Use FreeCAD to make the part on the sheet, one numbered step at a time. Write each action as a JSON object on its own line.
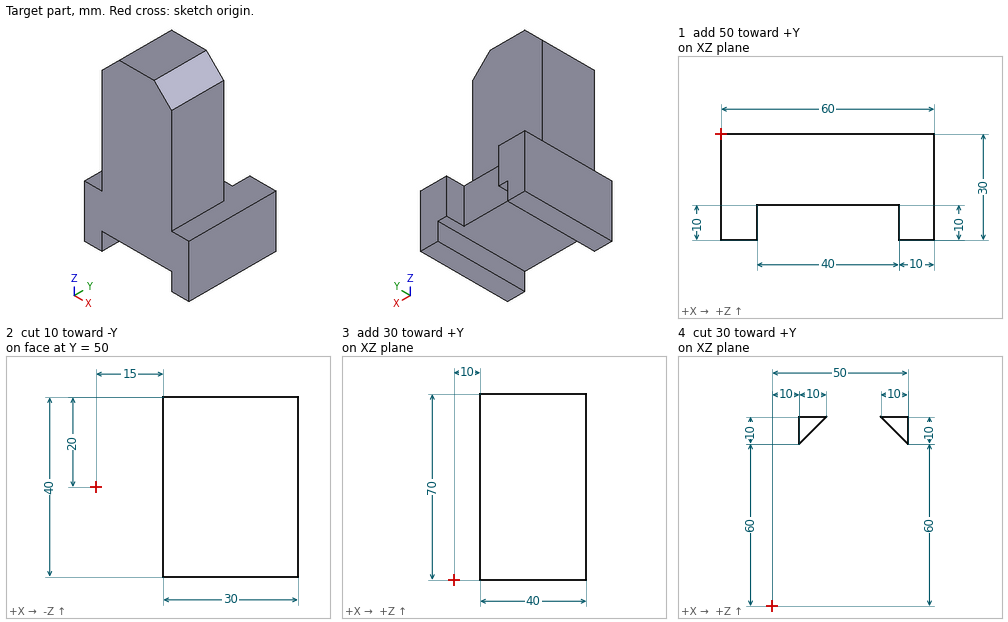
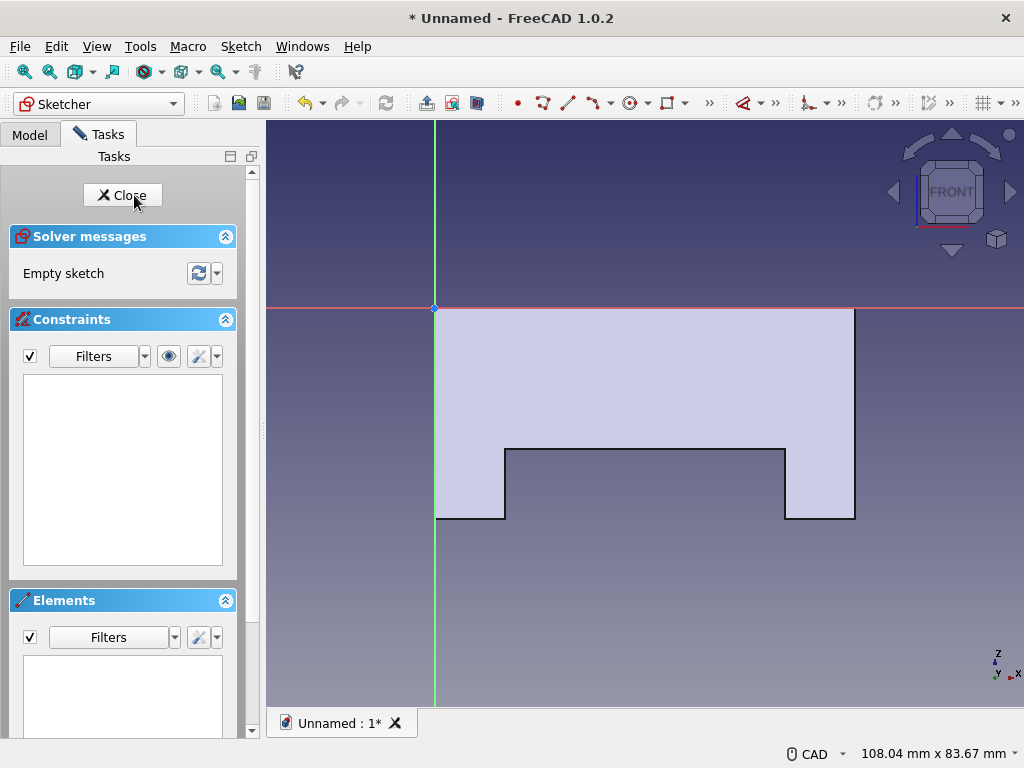
{"action": "scroll", "coordinate": [536, 679], "scroll_direction": "down", "scroll_amount": 3}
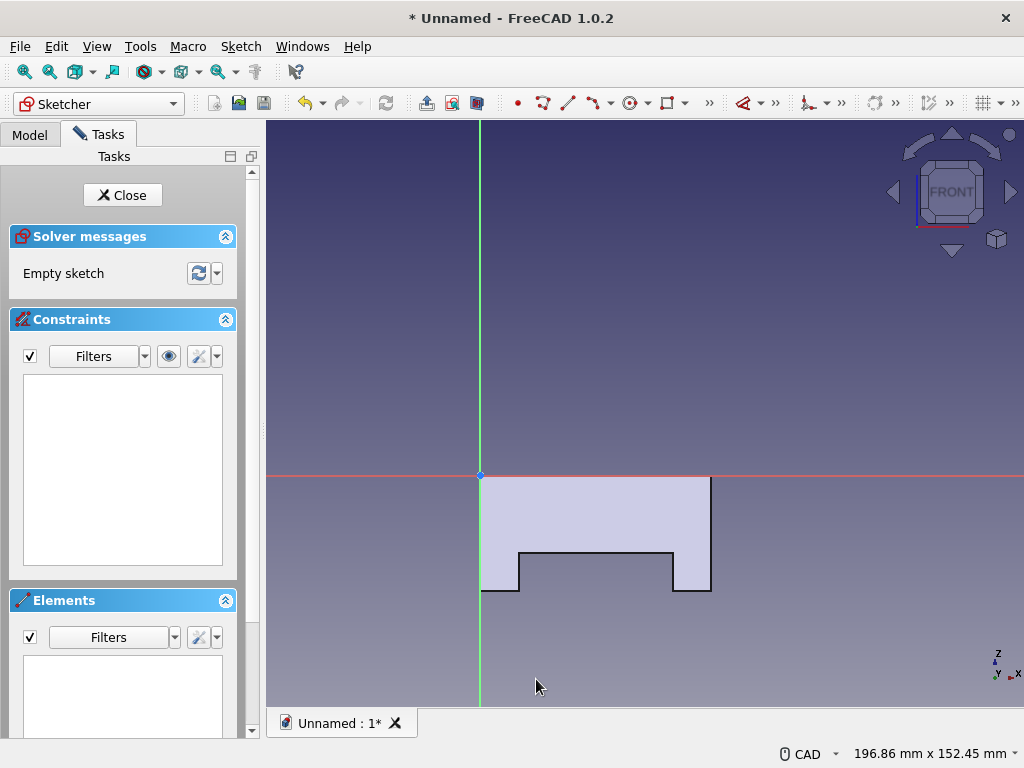
{"action": "scroll", "coordinate": [577, 194], "scroll_direction": "up", "scroll_amount": 2}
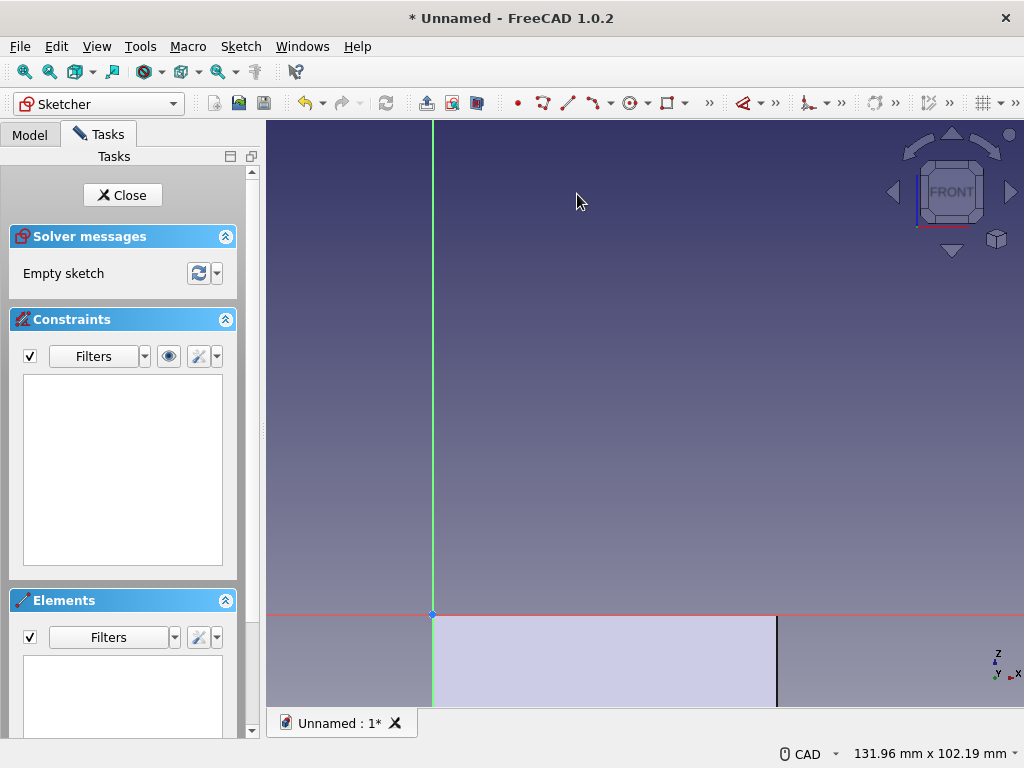
{"action": "key", "text": "g r"}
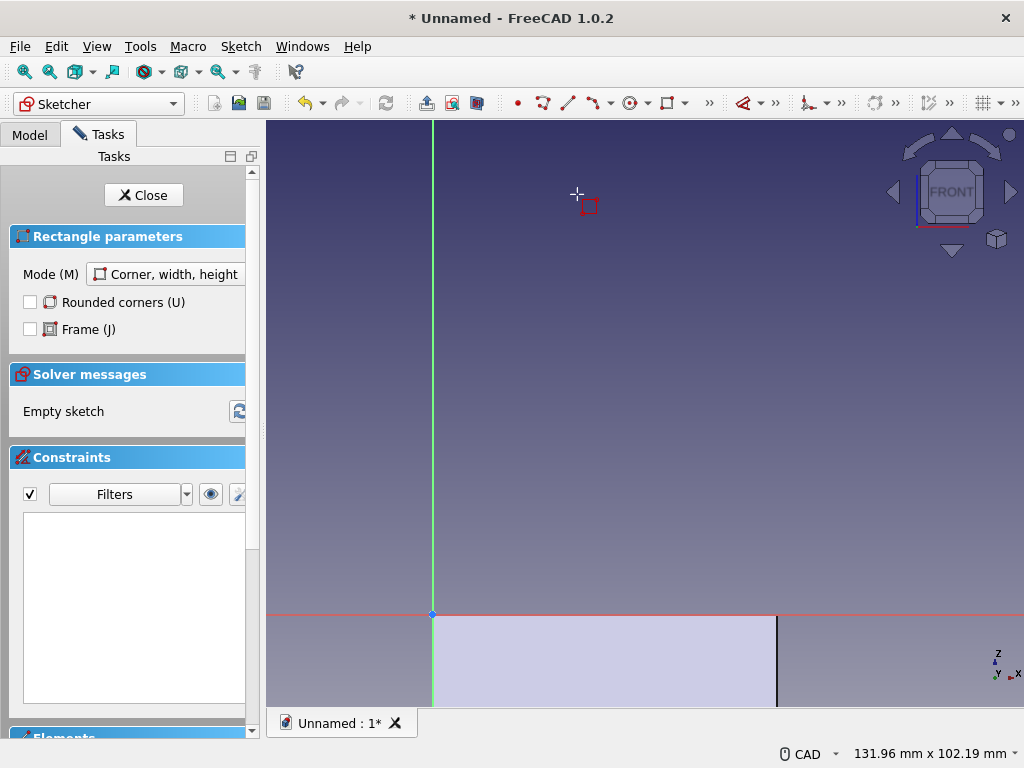
{"action": "left_click", "coordinate": [490, 212]}
{"action": "left_click", "coordinate": [720, 615]}
{"action": "key", "text": "Escape"}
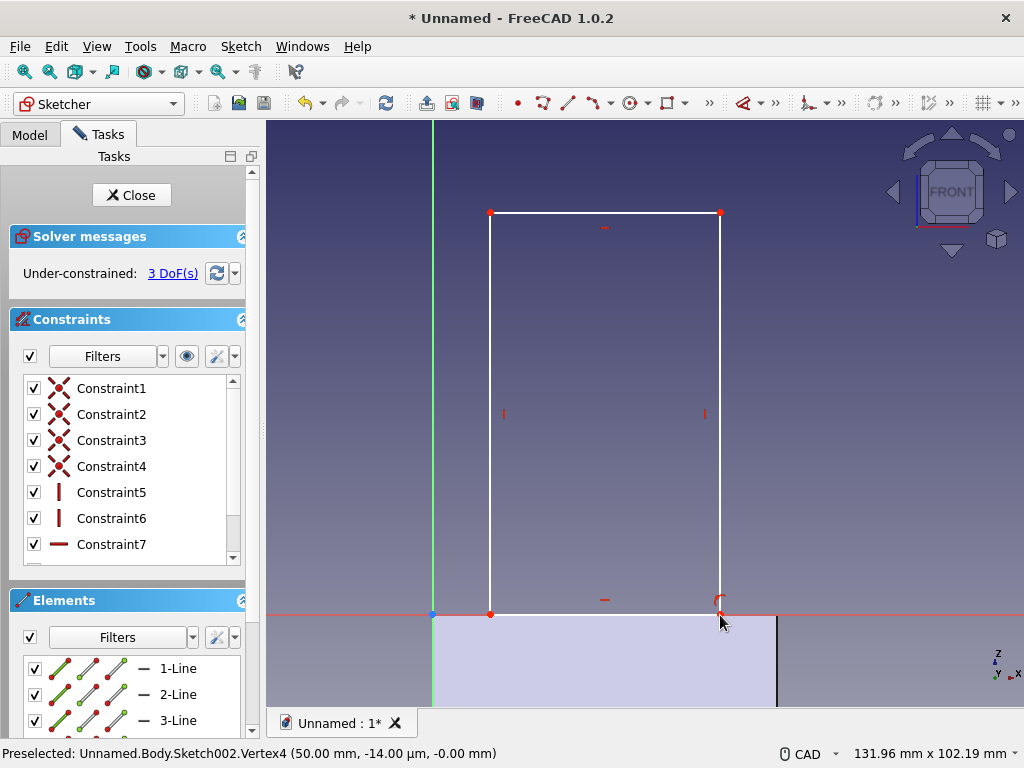
{"action": "key", "text": "d"}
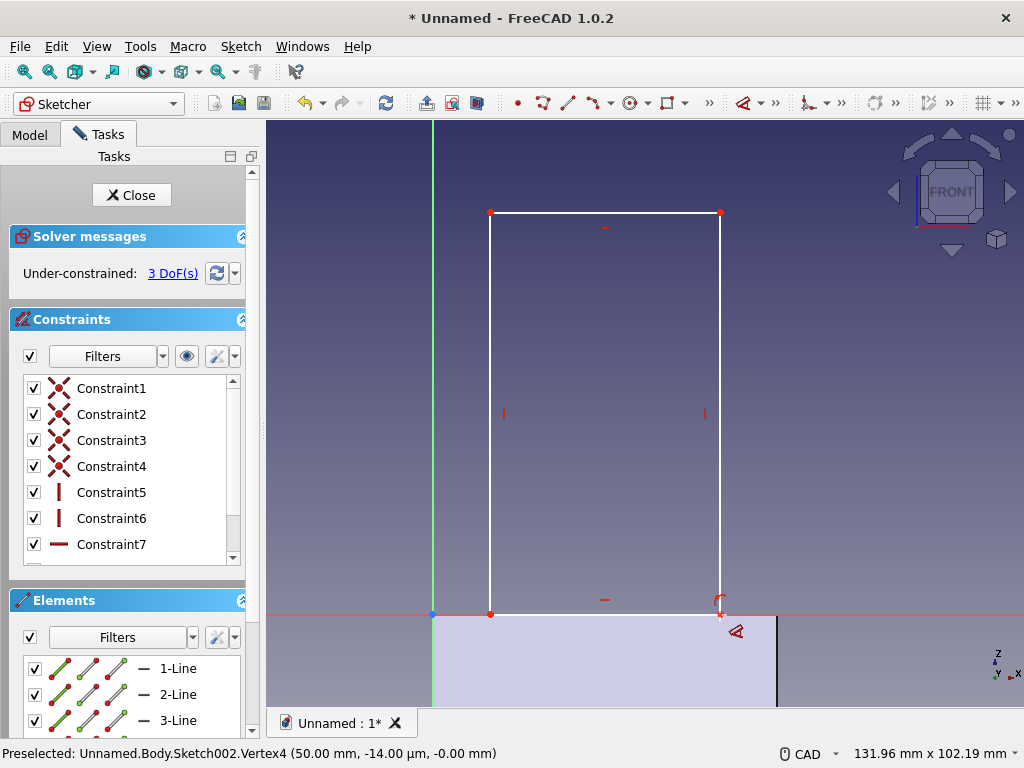
{"action": "left_click", "coordinate": [490, 333]}
{"action": "left_click", "coordinate": [456, 414]}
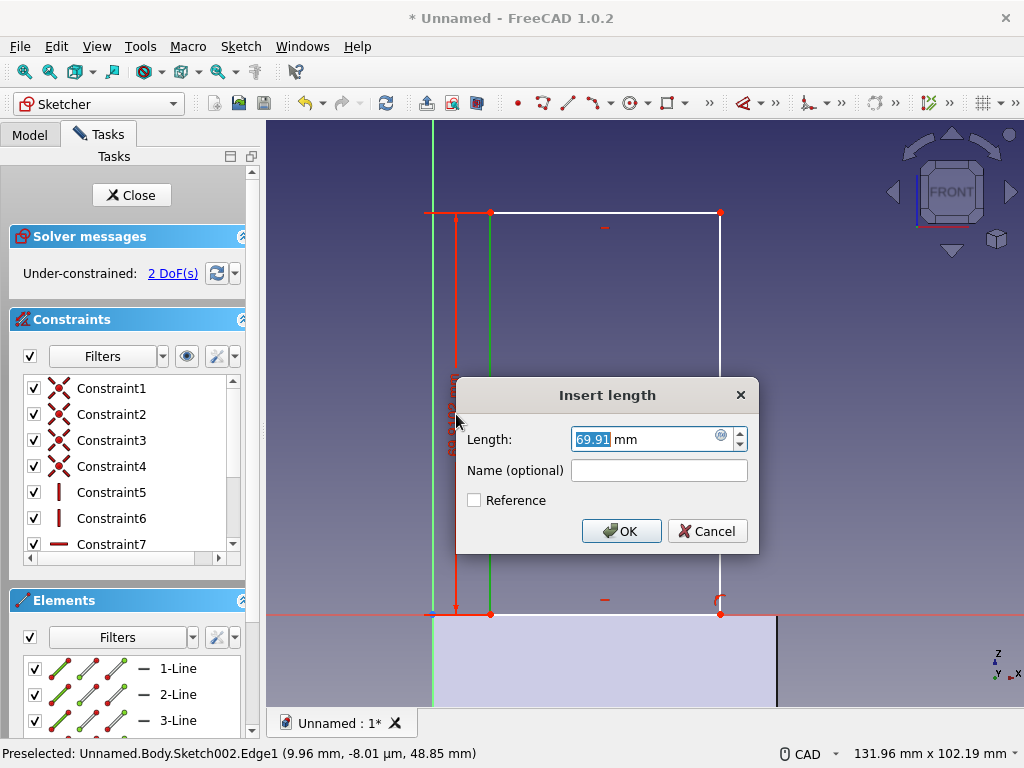
{"action": "type", "text": "70"}
{"action": "key", "text": "Return"}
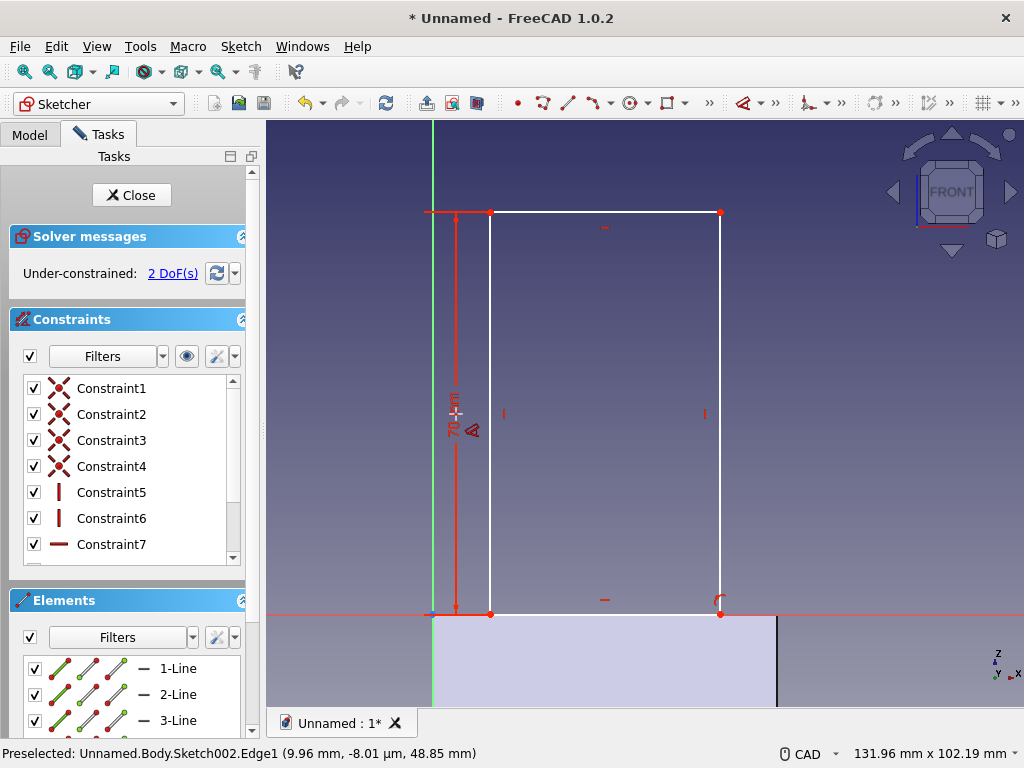
{"action": "left_click", "coordinate": [559, 615]}
{"action": "left_click", "coordinate": [605, 649]}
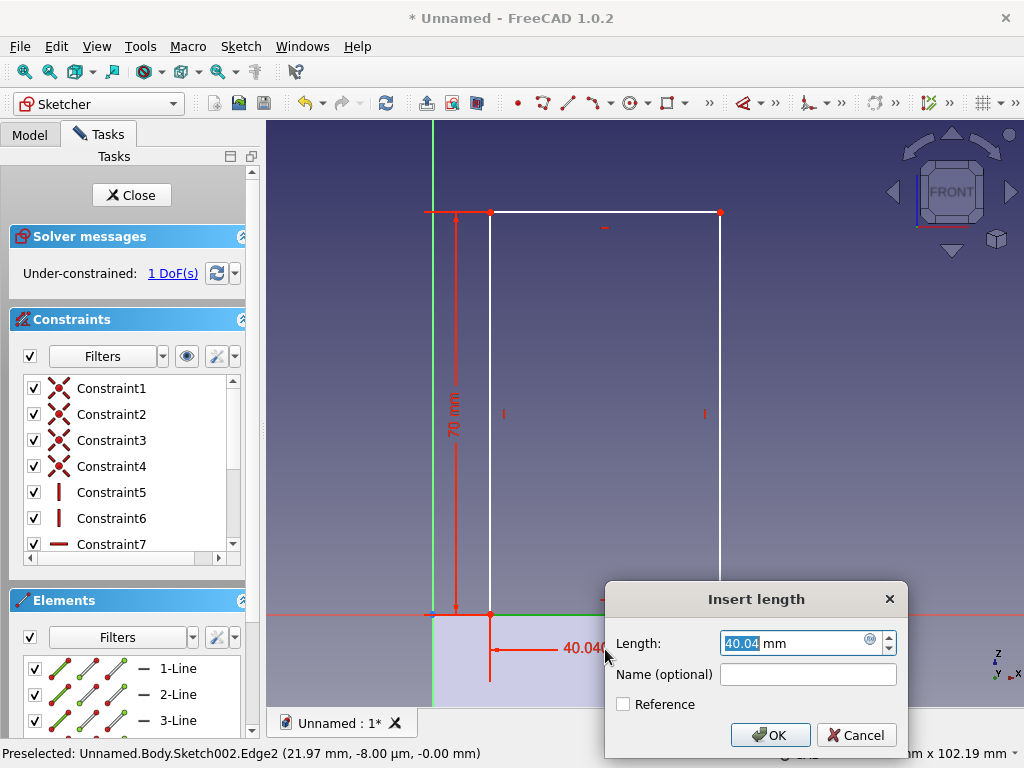
{"action": "type", "text": "40"}
{"action": "key", "text": "Return"}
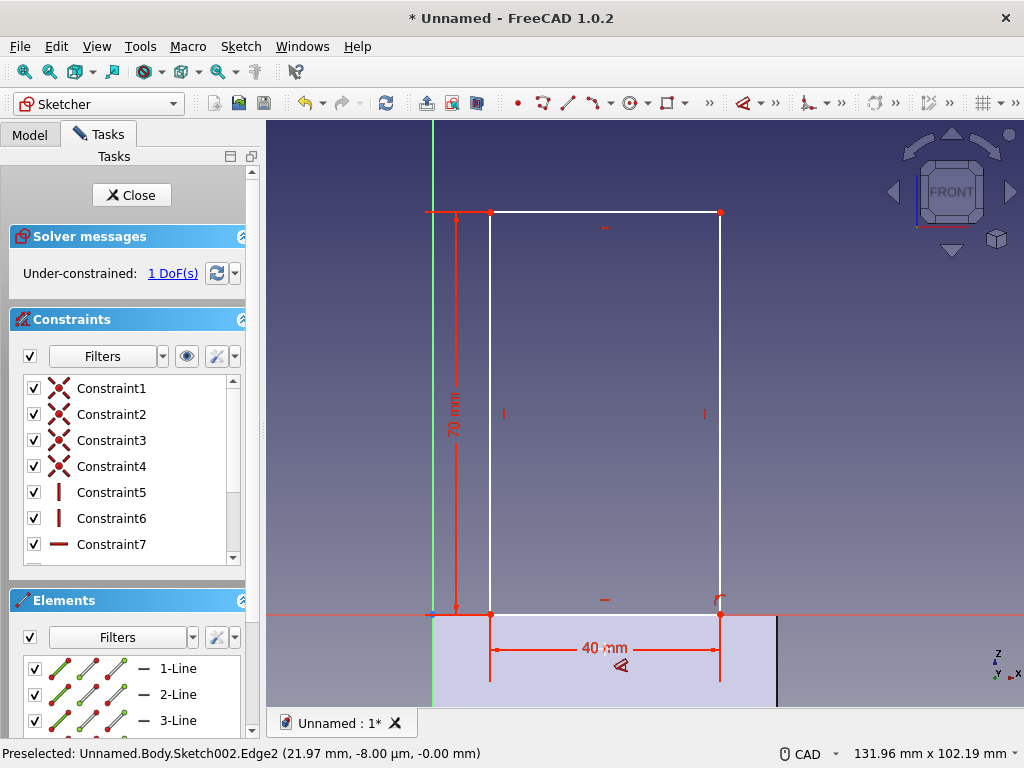
{"action": "left_click", "coordinate": [490, 212]}
{"action": "left_click", "coordinate": [462, 649]}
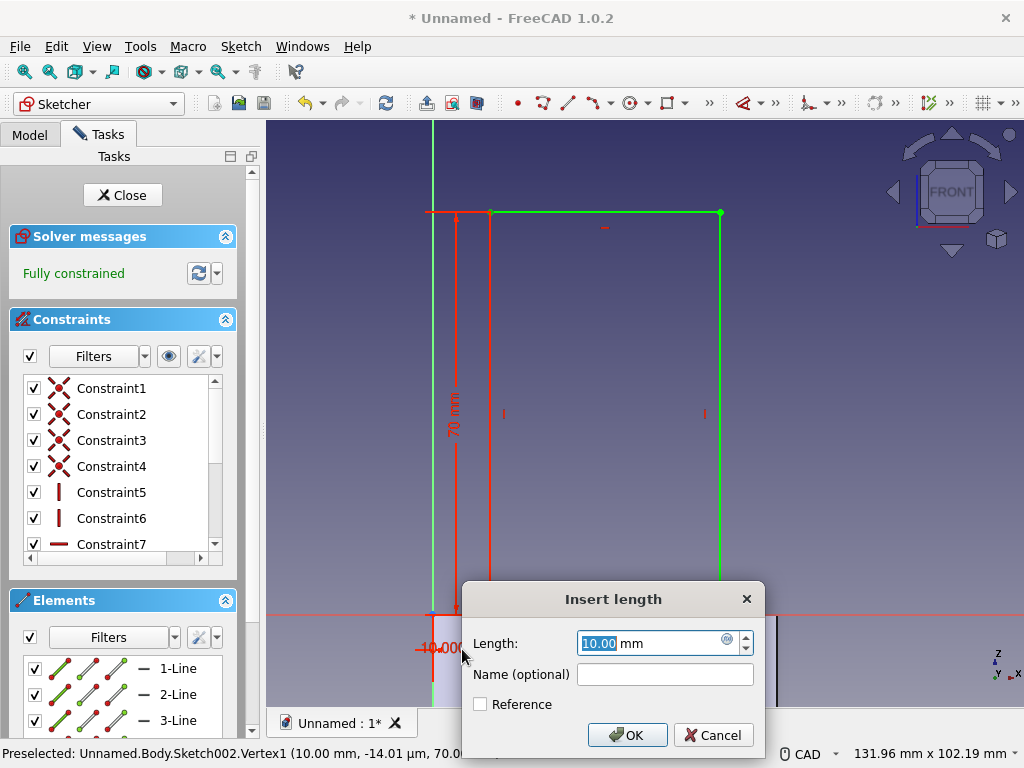
{"action": "type", "text": "10"}
{"action": "key", "text": "Return"}
{"action": "key", "text": "Escape"}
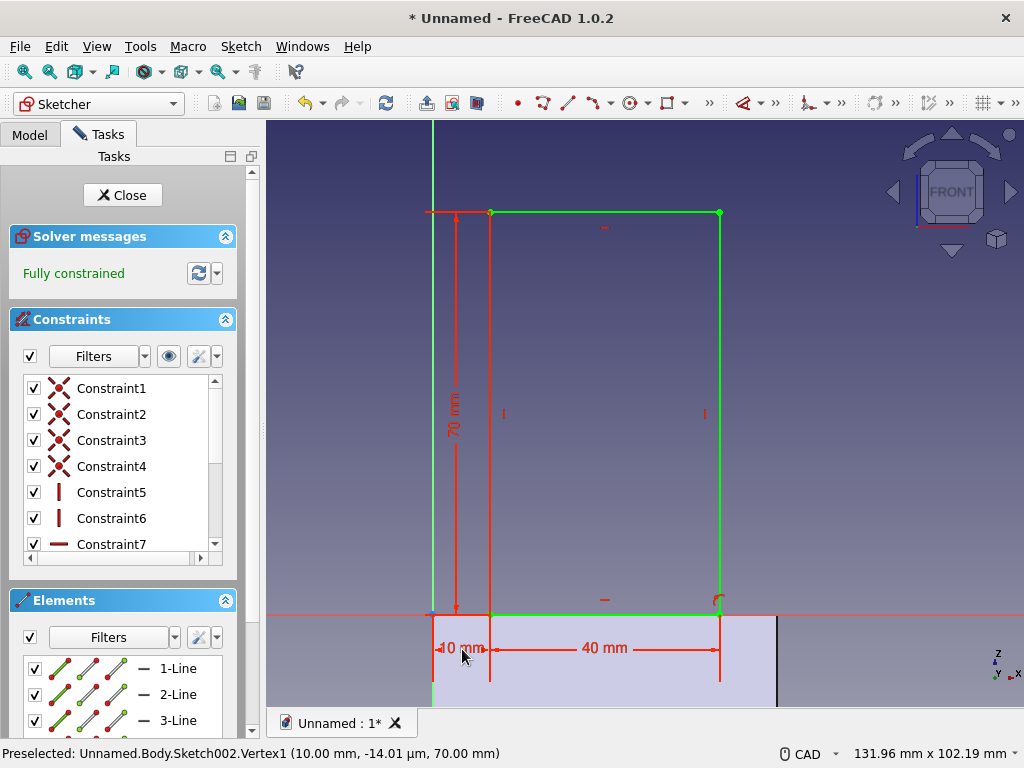
{"action": "left_click", "coordinate": [123, 195]}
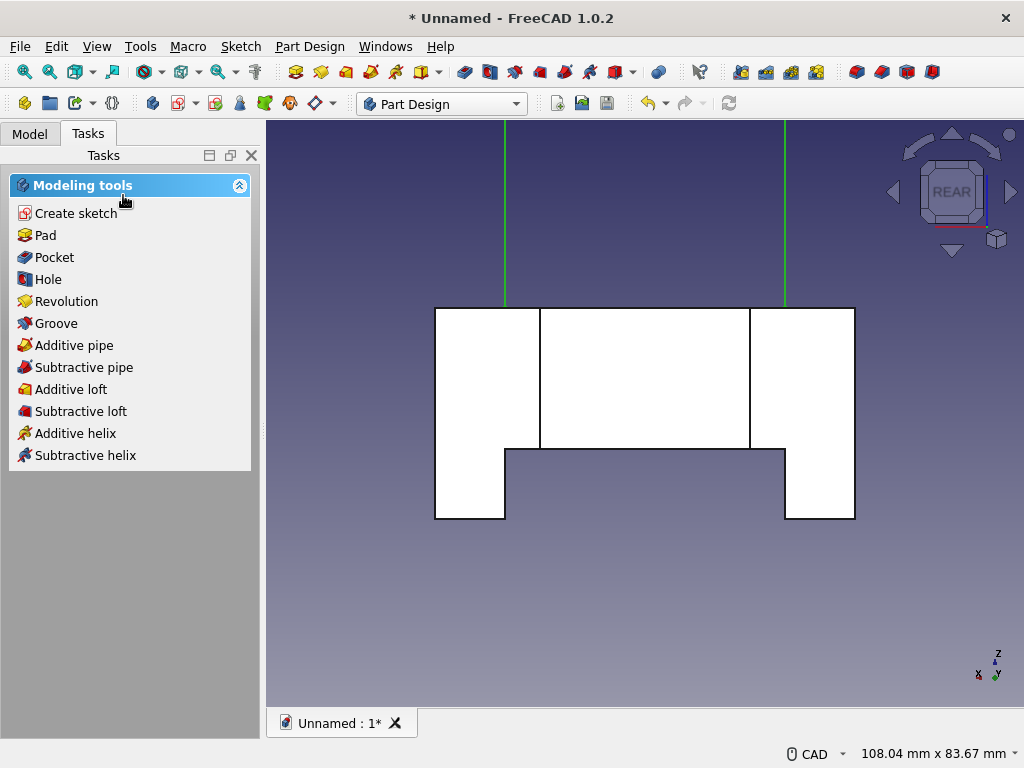
{"action": "left_click", "coordinate": [296, 72]}